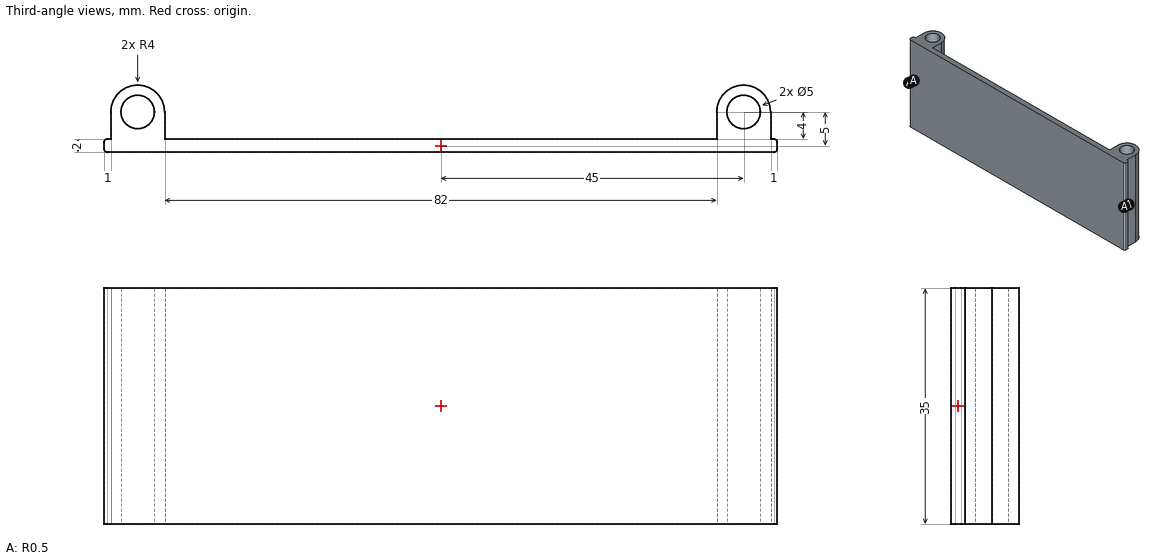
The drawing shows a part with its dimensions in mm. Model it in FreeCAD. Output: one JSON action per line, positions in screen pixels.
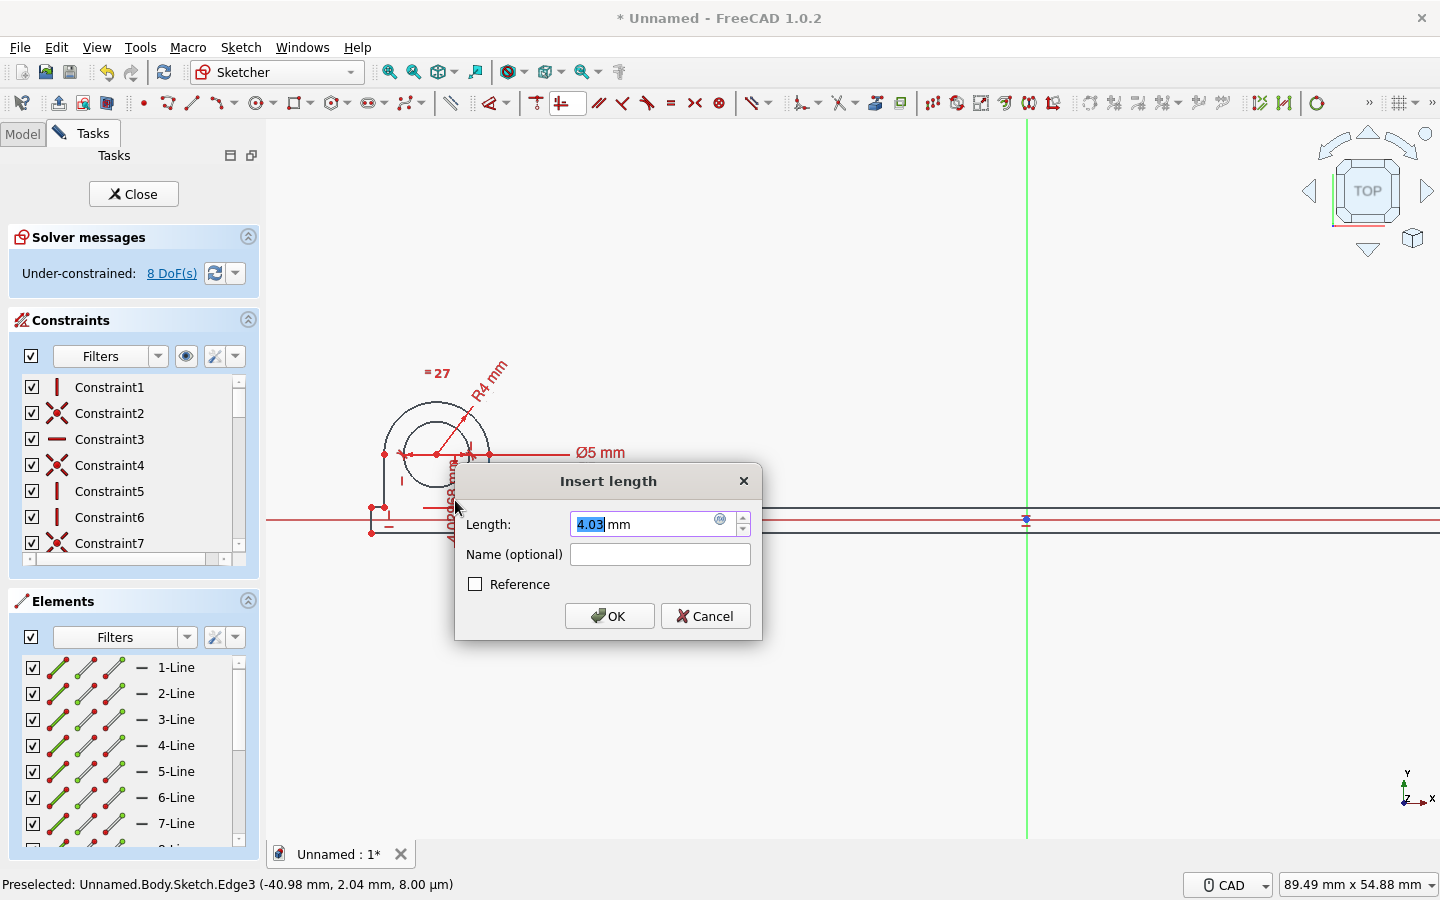
{"action": "type", "text": "4"}
{"action": "key", "text": "Return"}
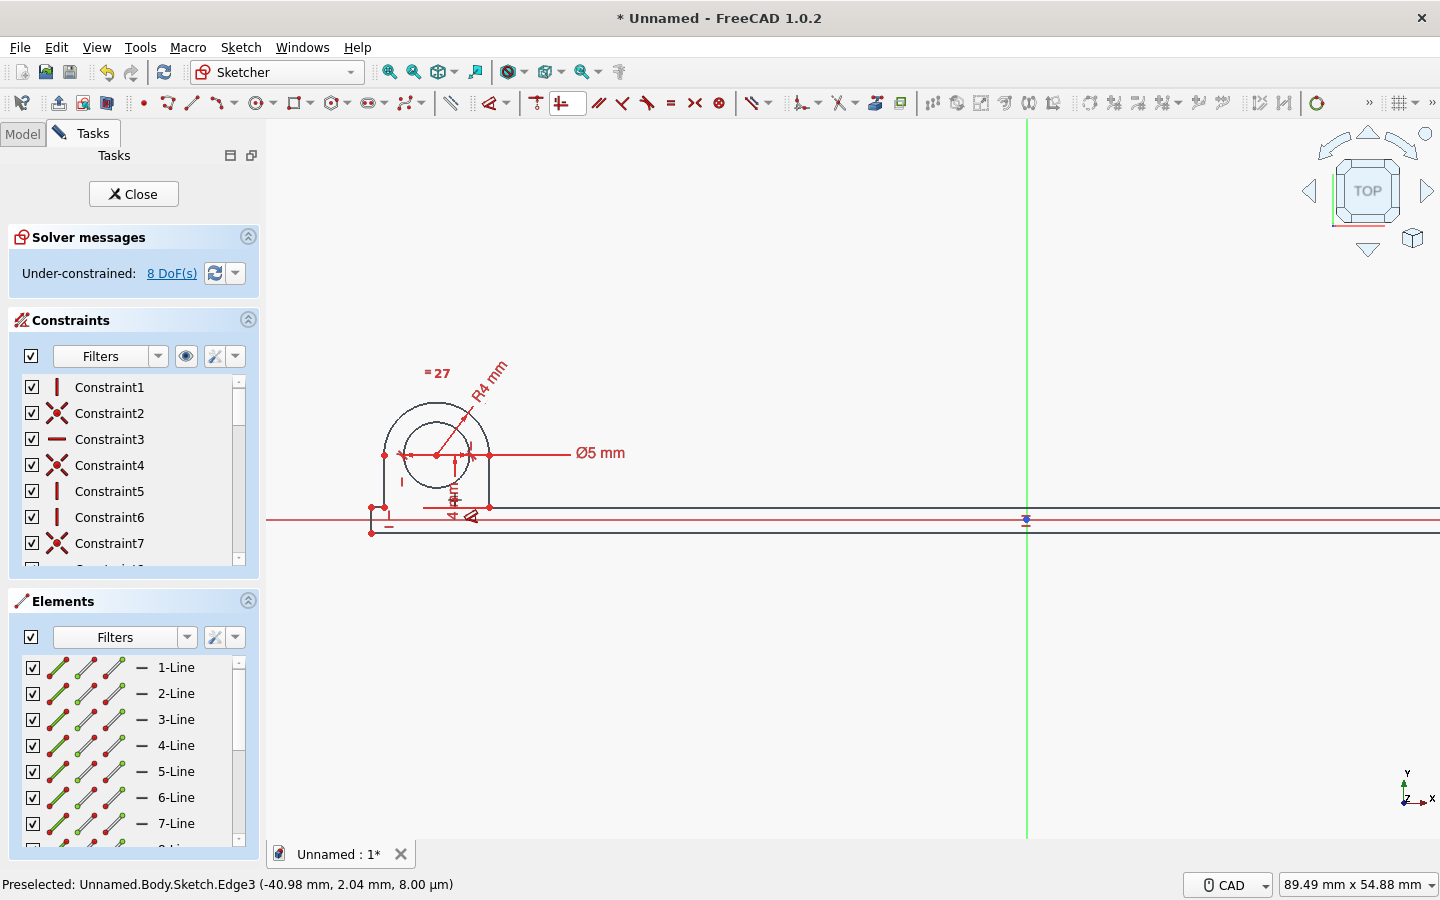
{"action": "left_click", "coordinate": [384, 471]}
{"action": "left_click", "coordinate": [350, 481]}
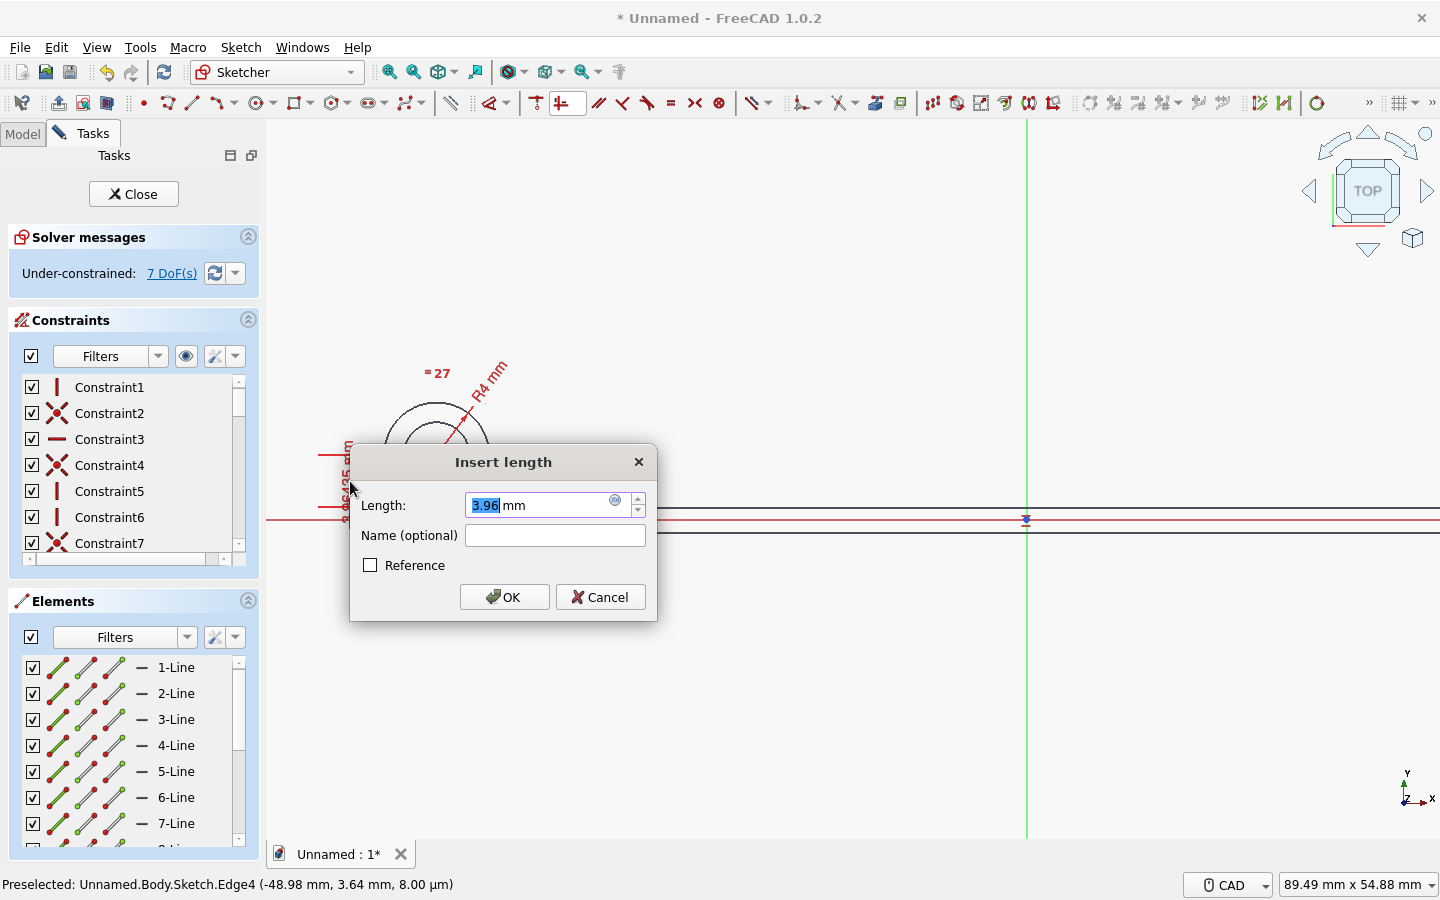
{"action": "type", "text": "4"}
{"action": "key", "text": "Return"}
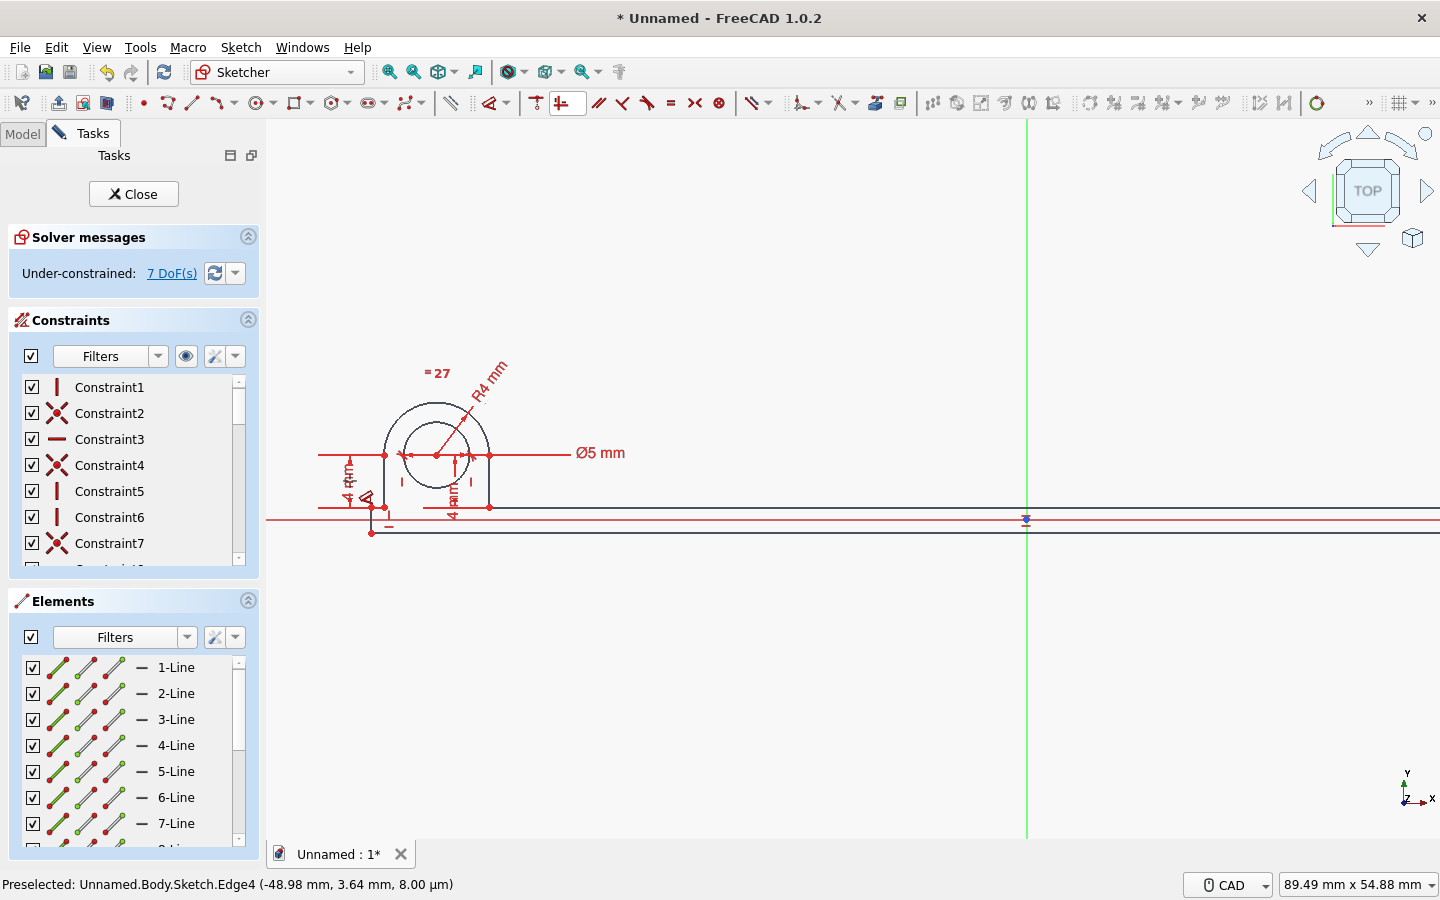
{"action": "scroll", "coordinate": [378, 508], "scroll_direction": "up", "scroll_amount": 6}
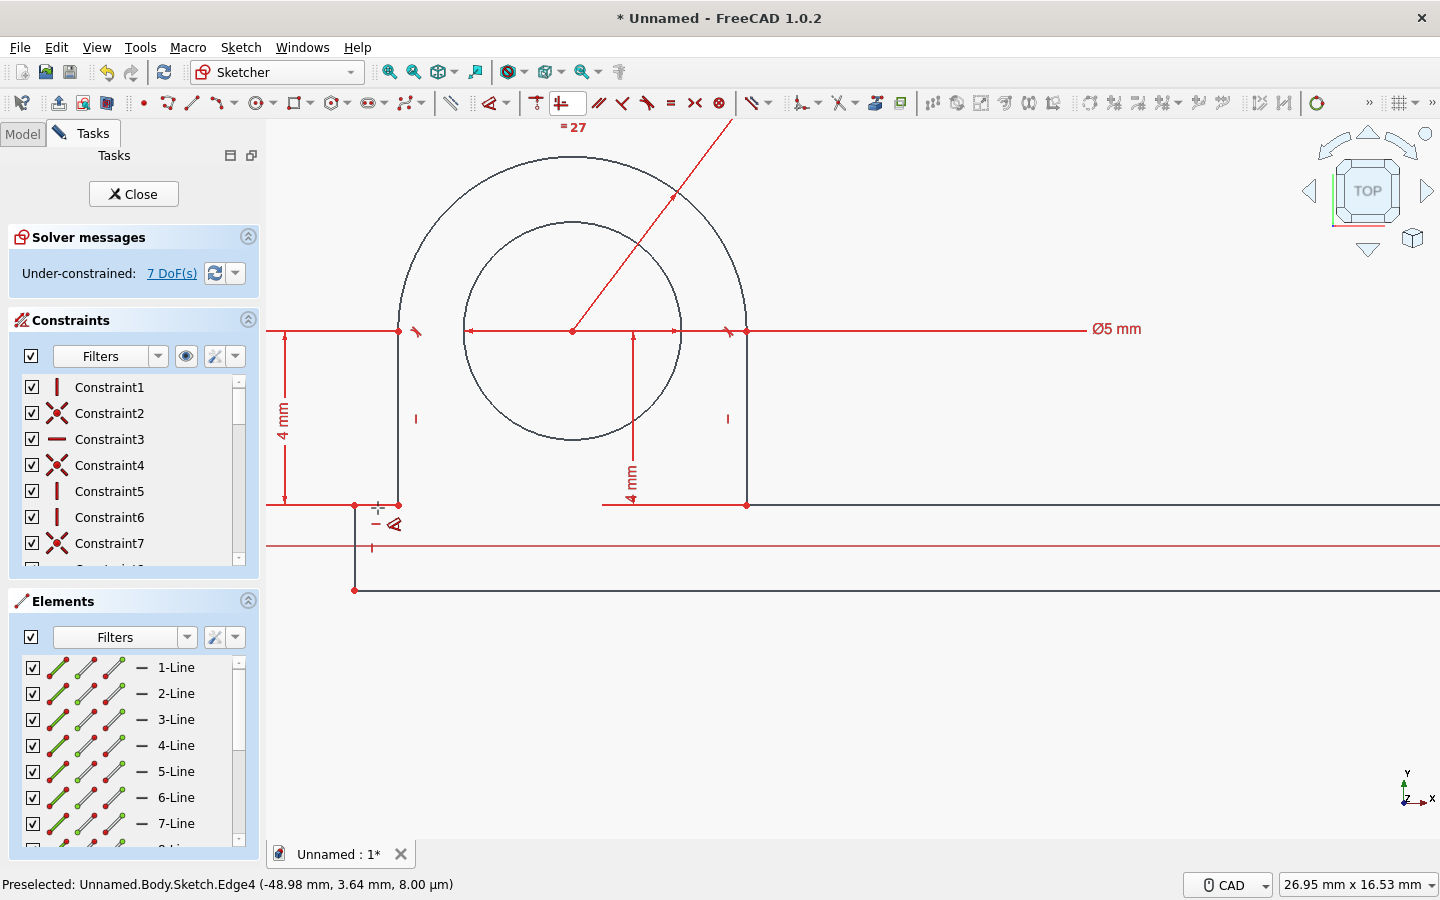
{"action": "left_click", "coordinate": [377, 505]}
{"action": "left_click", "coordinate": [377, 471]}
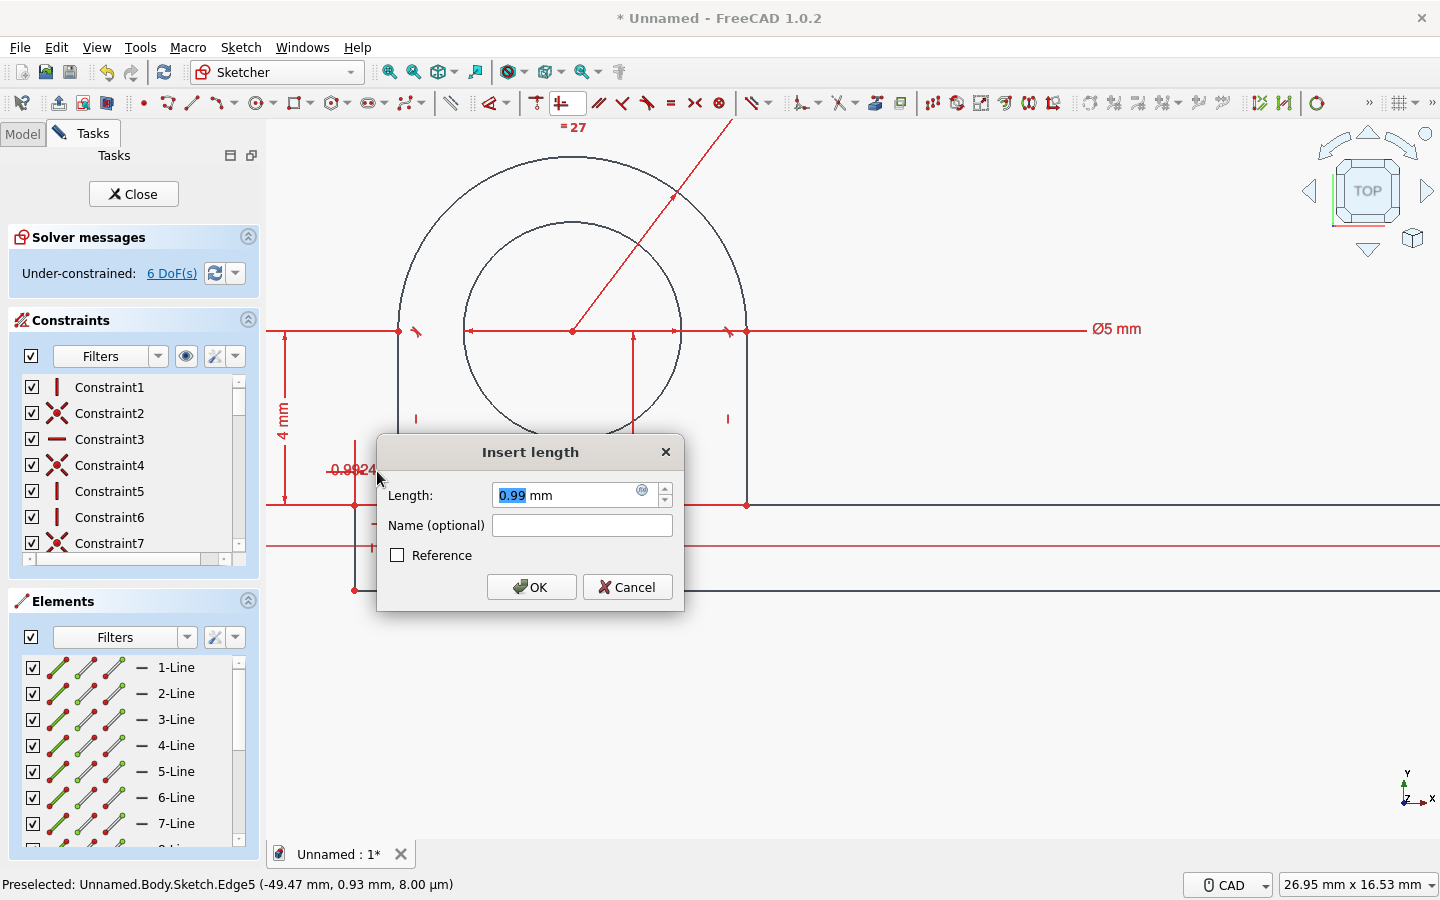
{"action": "type", "text": "1"}
{"action": "key", "text": "Return"}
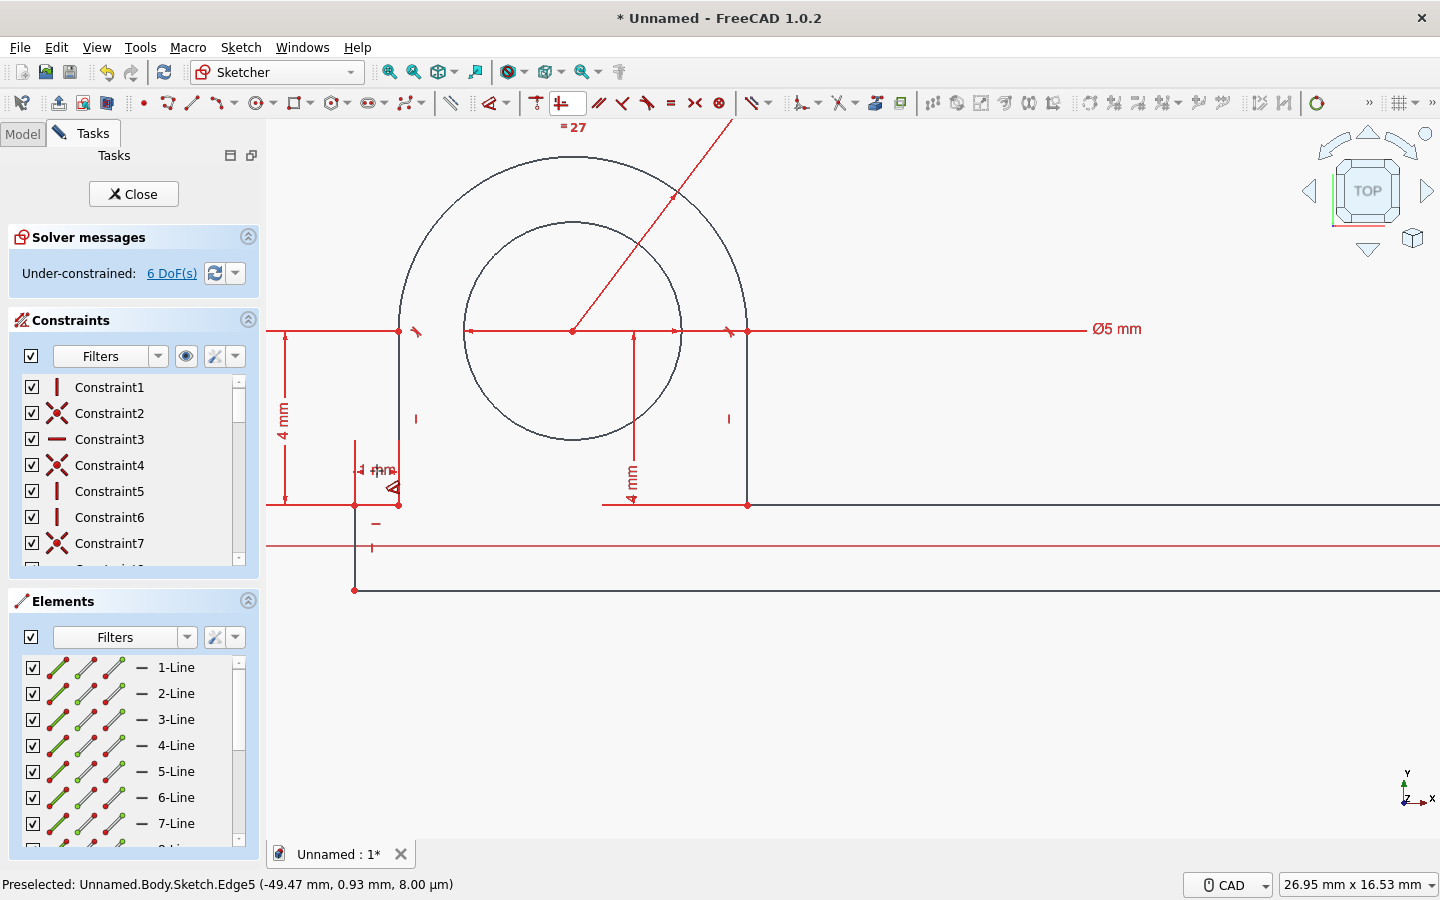
{"action": "left_click", "coordinate": [355, 531]}
{"action": "left_click", "coordinate": [321, 528]}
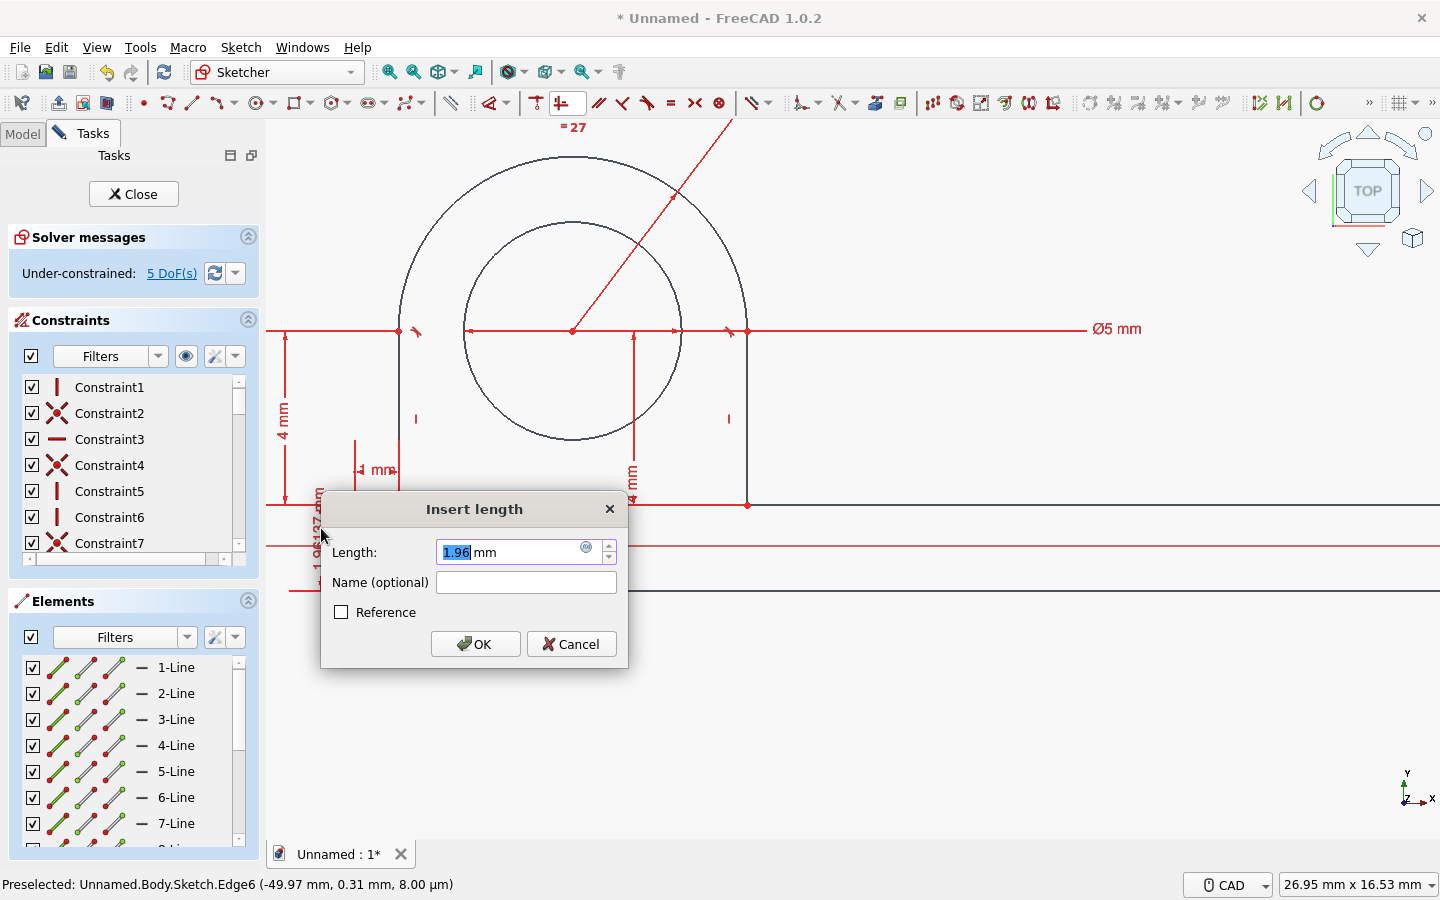
{"action": "type", "text": "2"}
{"action": "key", "text": "Return"}